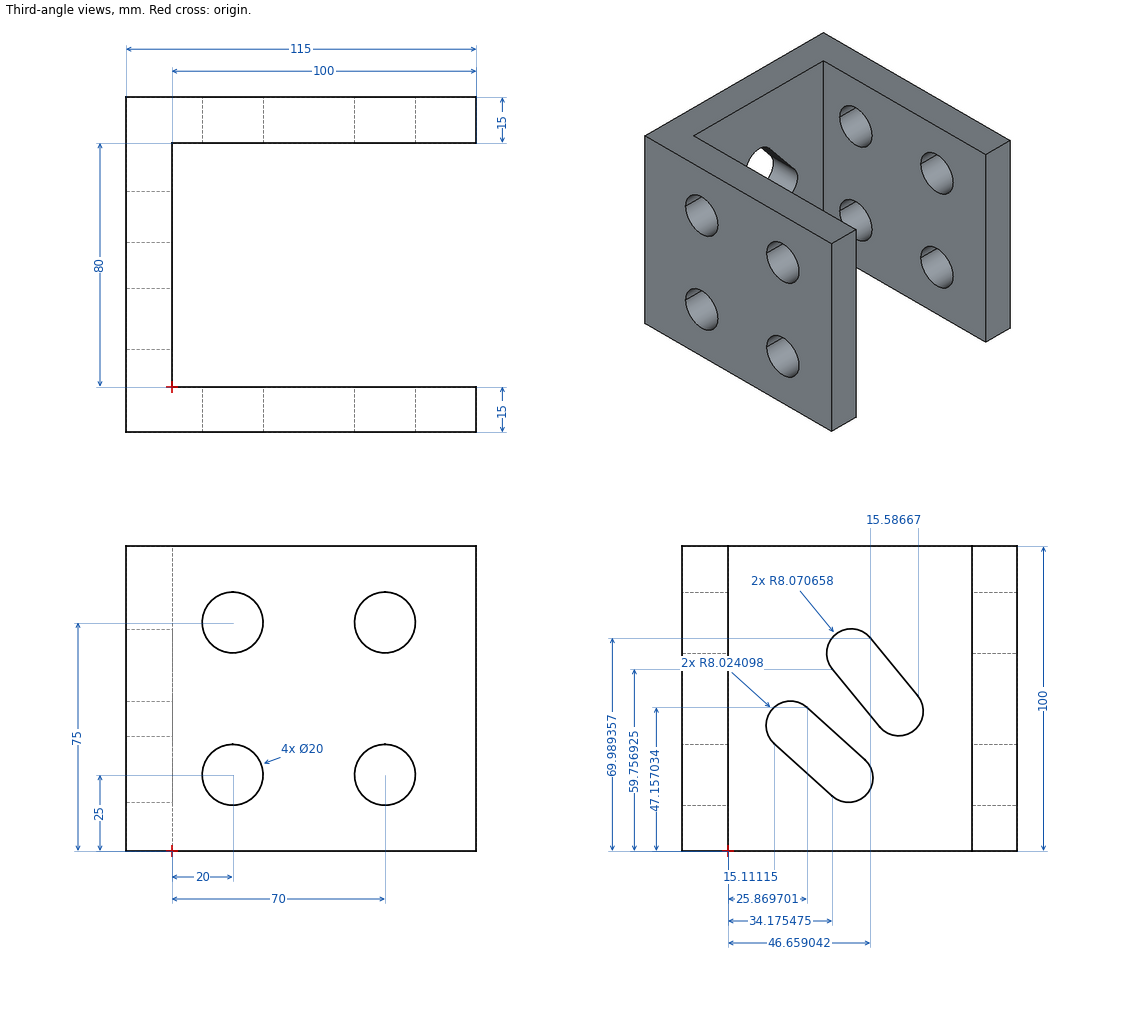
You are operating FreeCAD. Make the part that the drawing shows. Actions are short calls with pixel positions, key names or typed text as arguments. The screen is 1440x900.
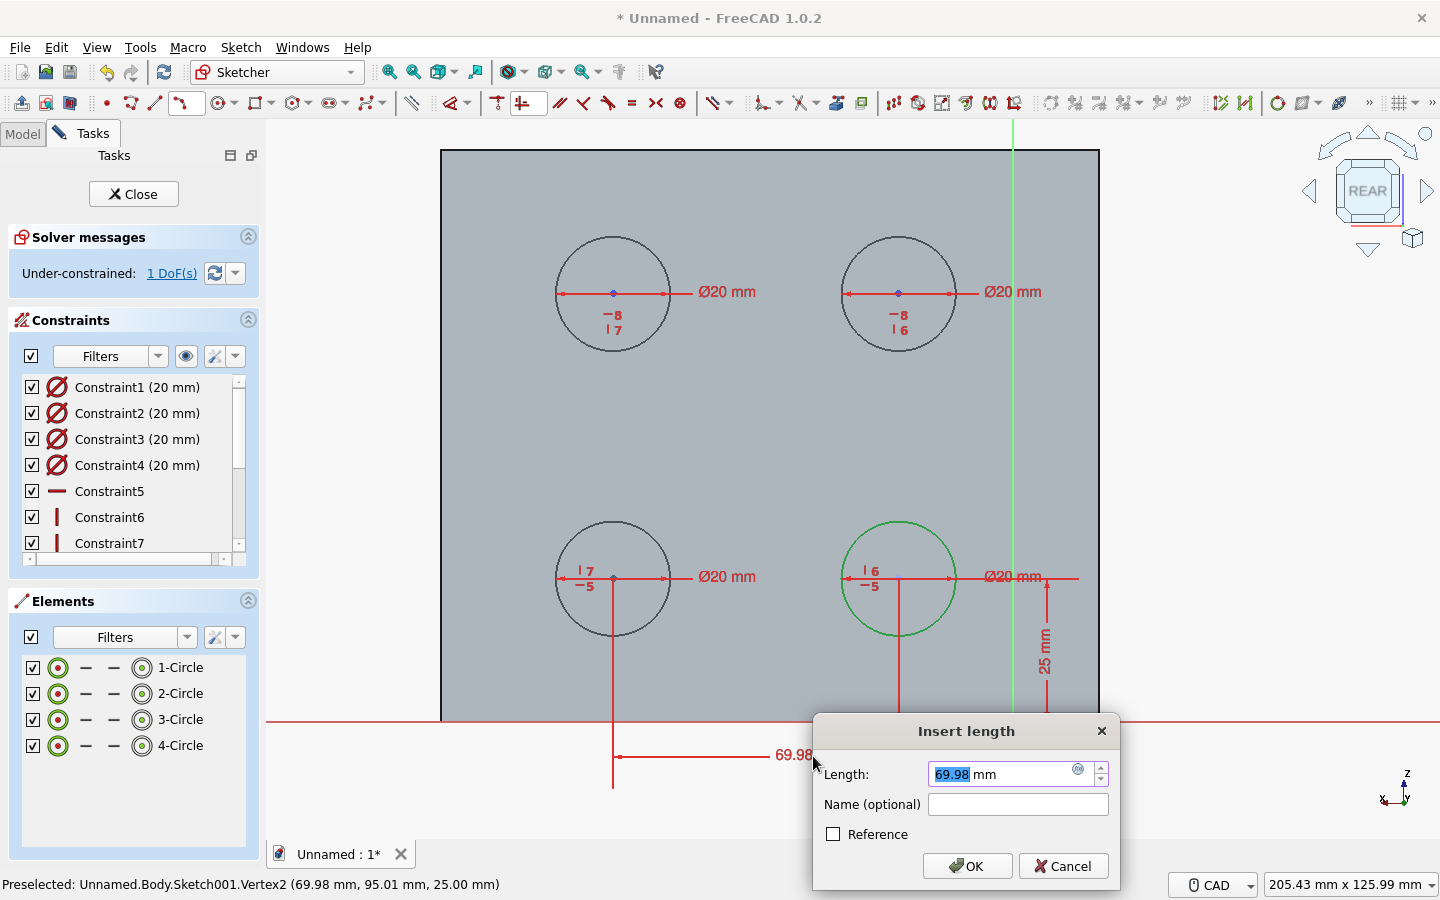
text(70)
key(Return)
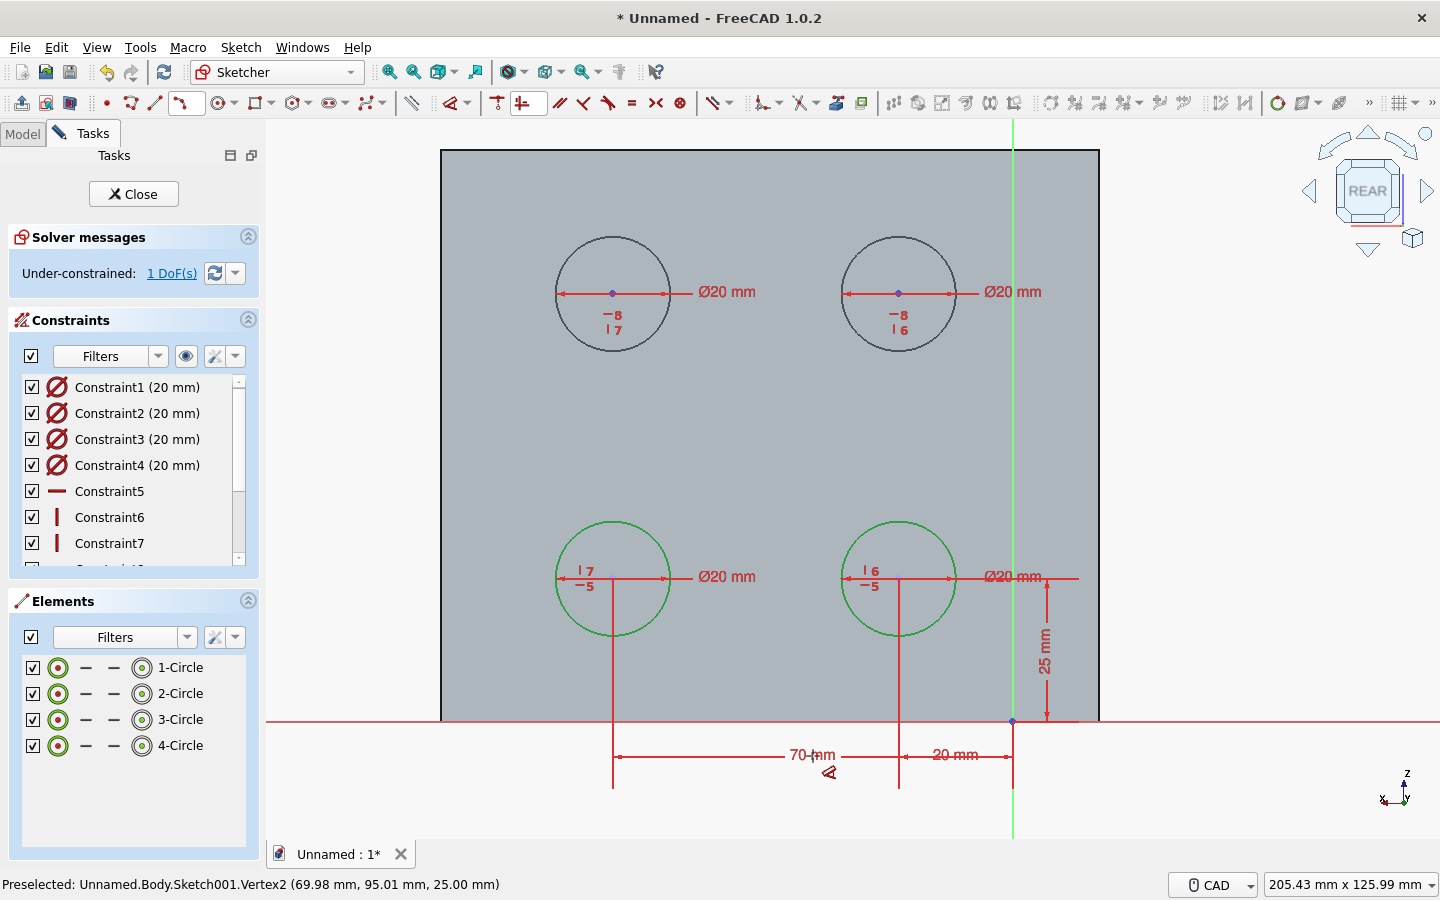
click(899, 294)
click(1047, 508)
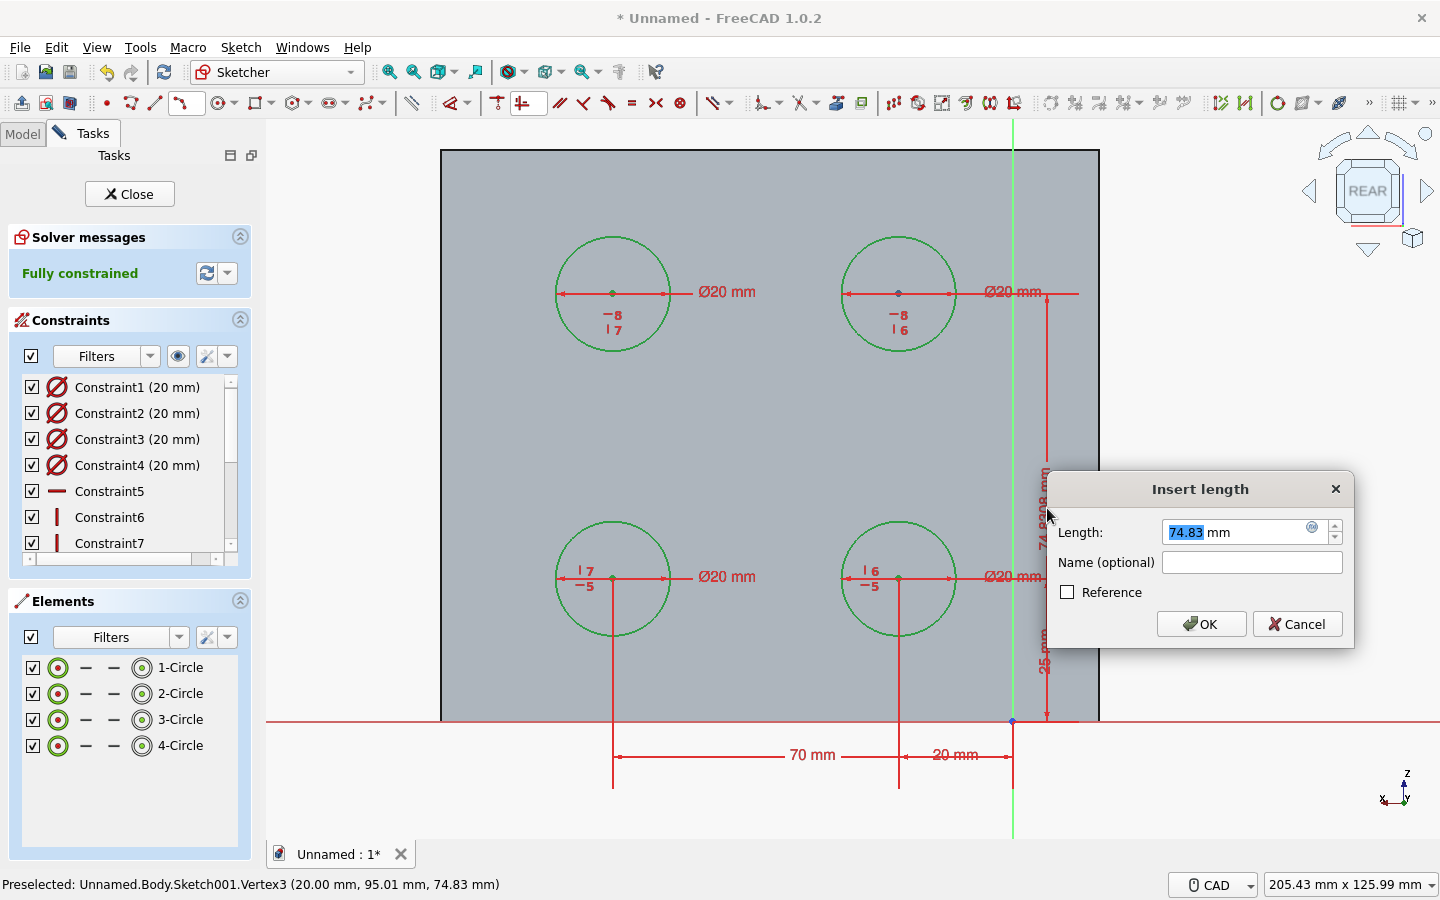
text(75)
key(Return)
key(Escape)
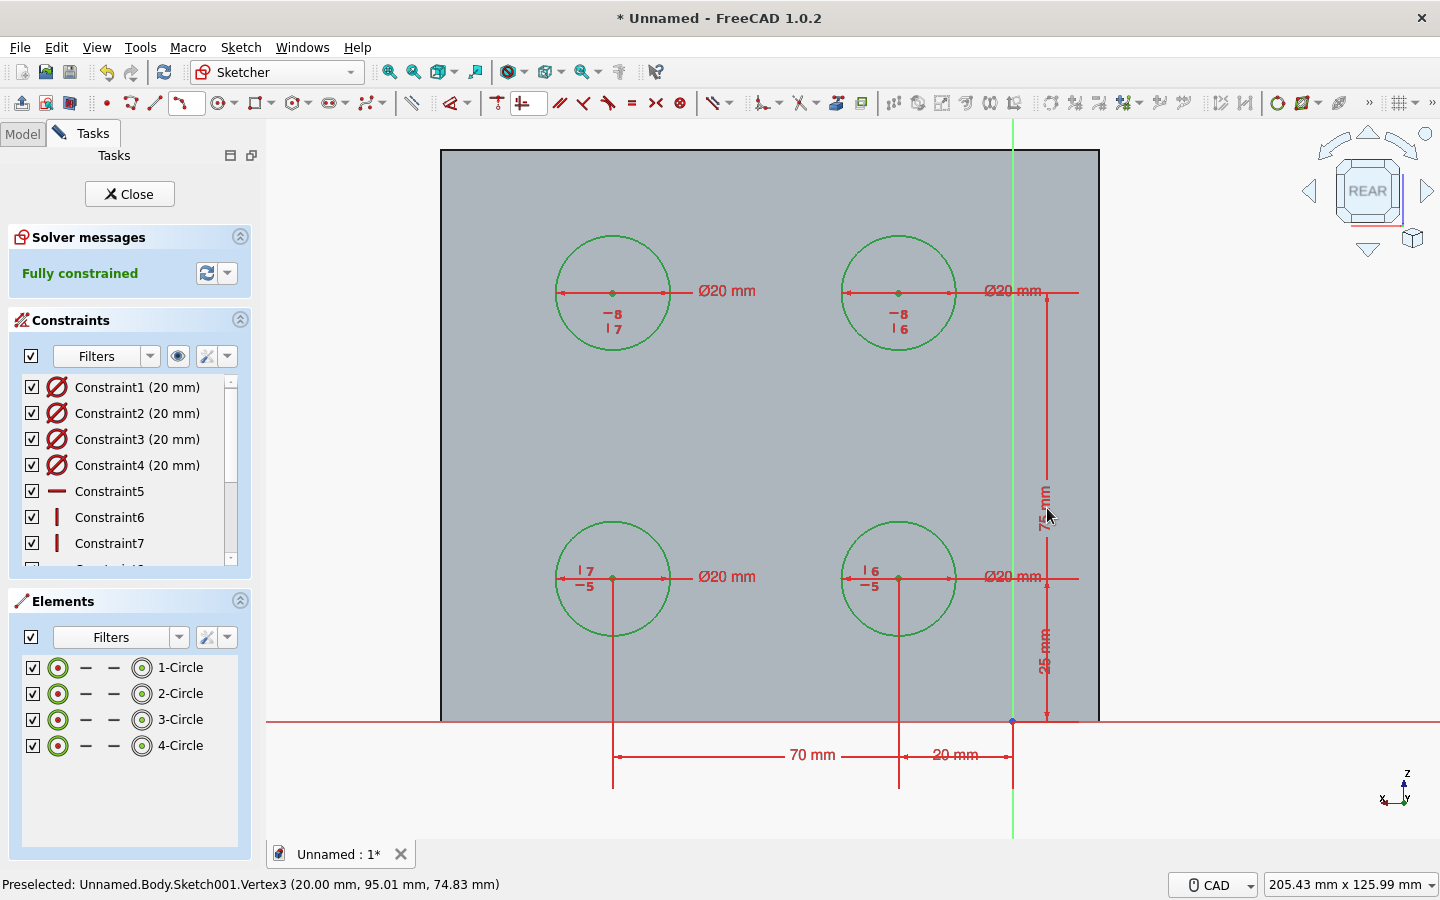
click(130, 194)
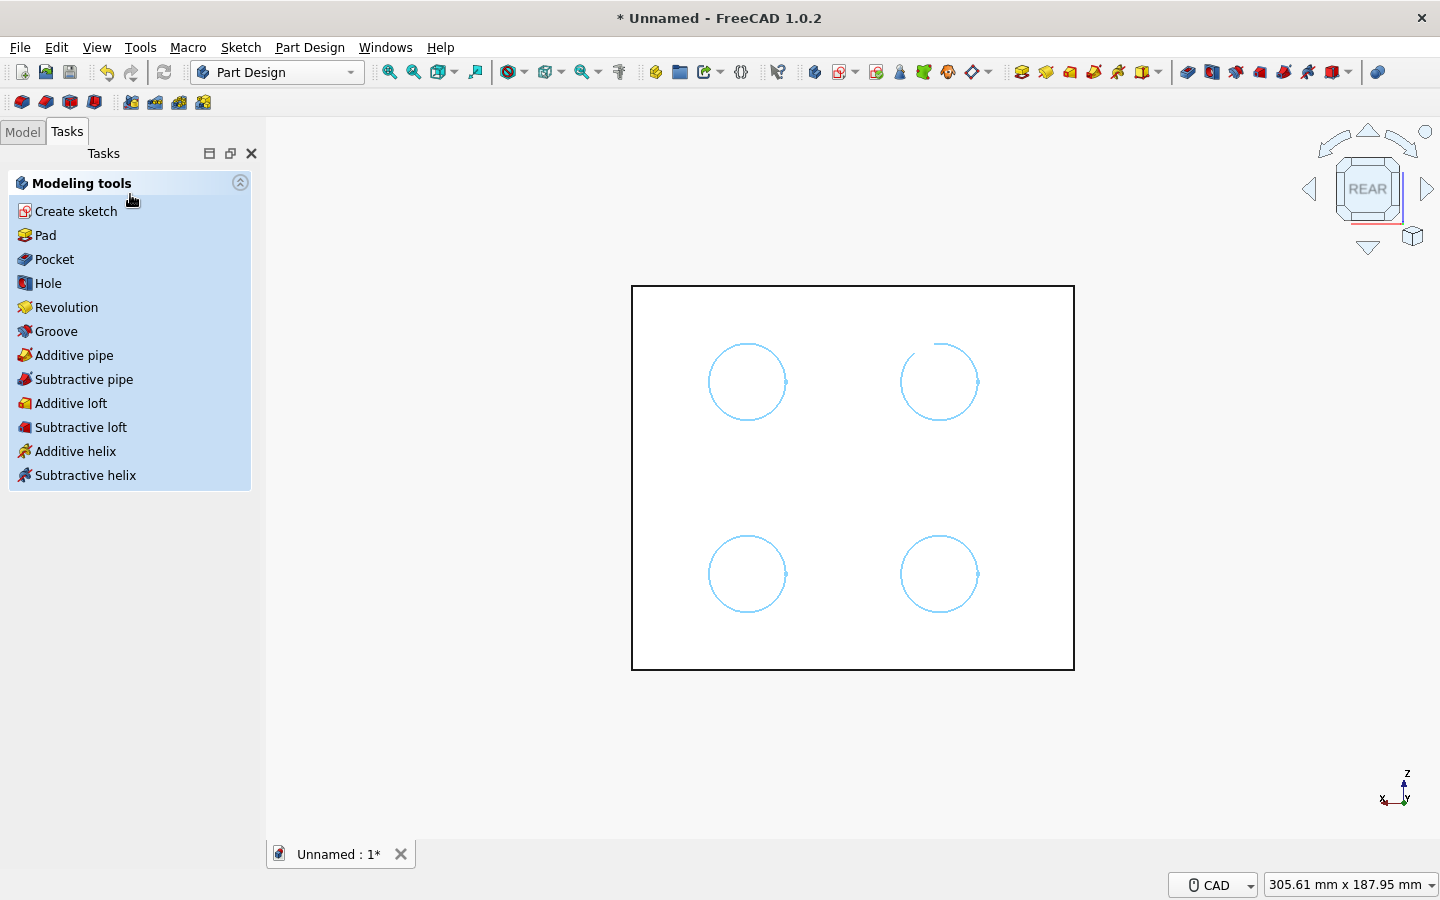
click(1188, 72)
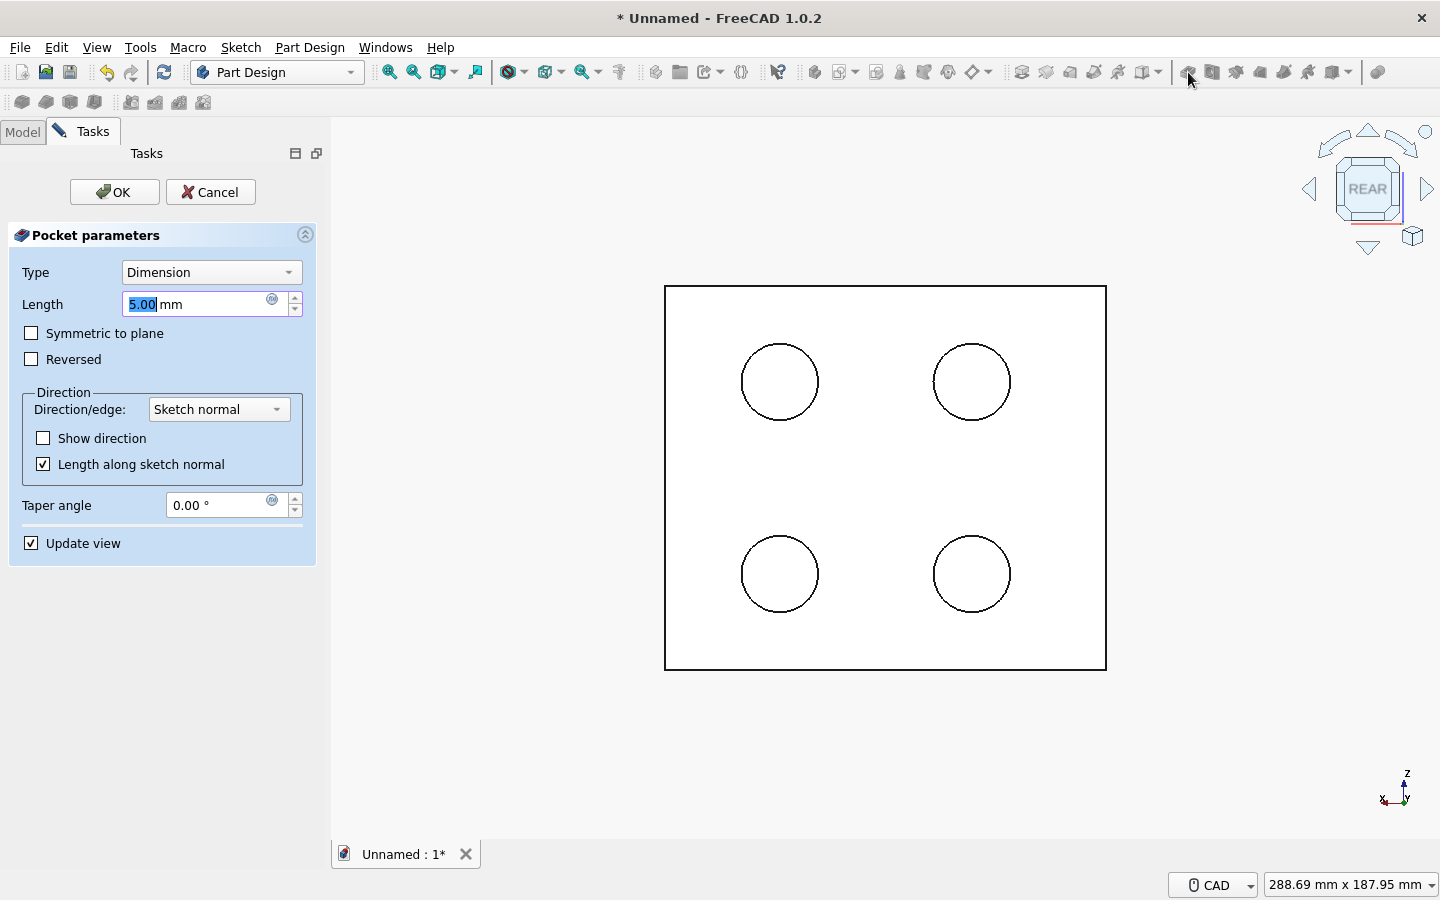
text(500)
key(Tab)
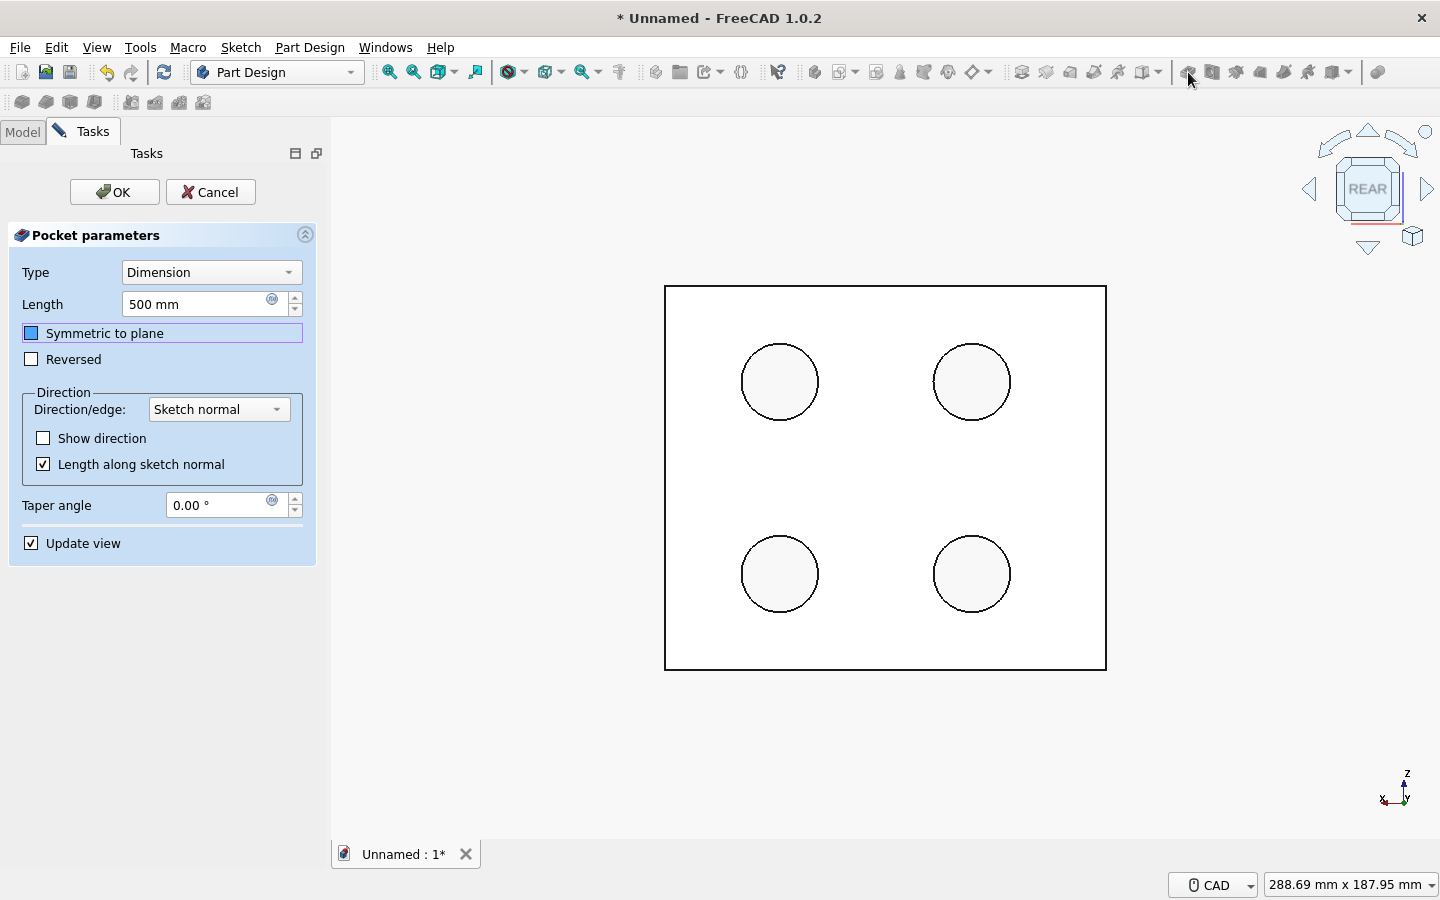
click(115, 192)